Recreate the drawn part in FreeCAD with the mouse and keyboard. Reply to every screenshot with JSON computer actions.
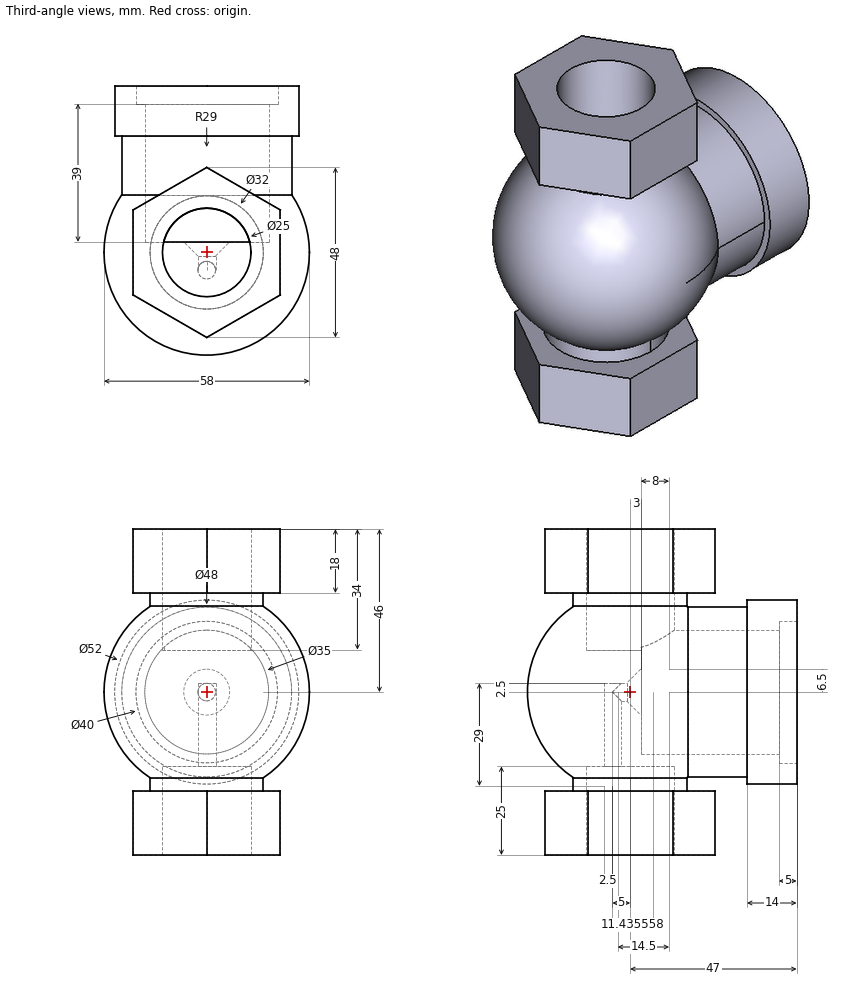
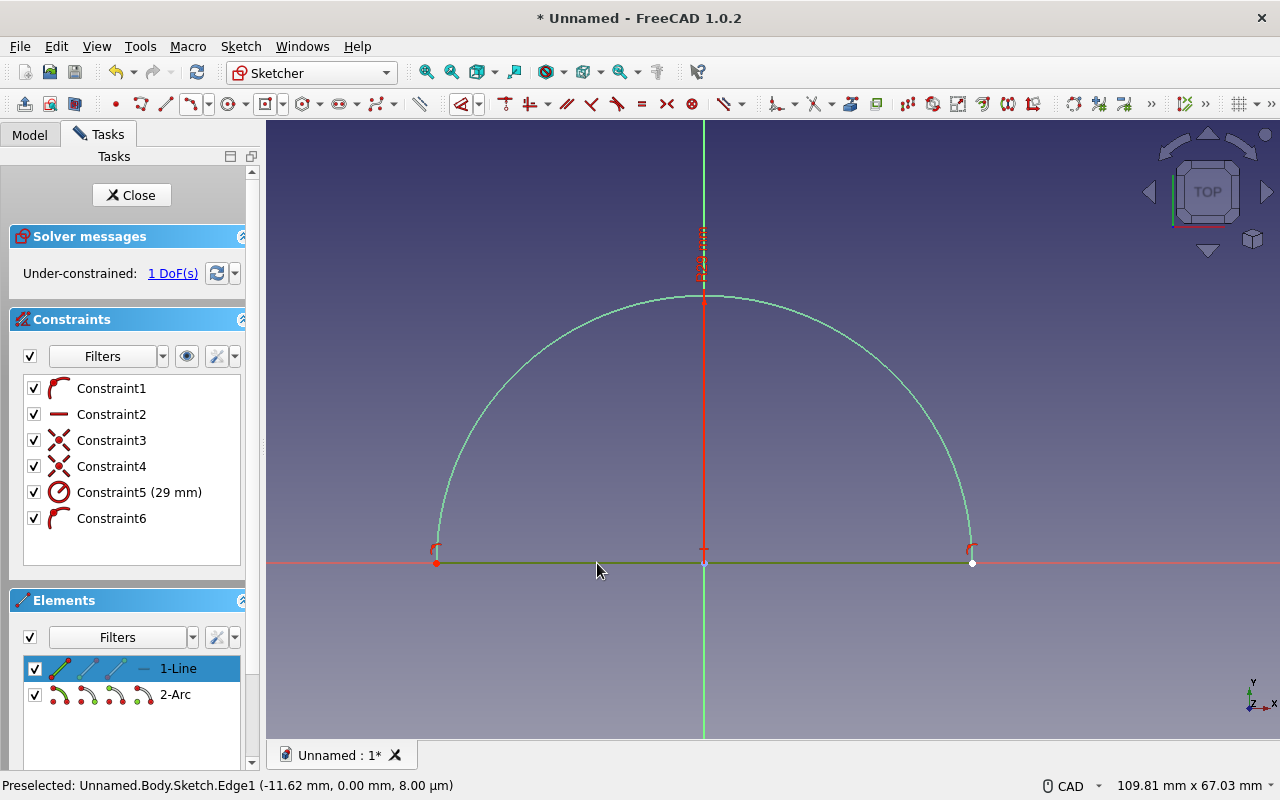
{"action": "key", "text": "l"}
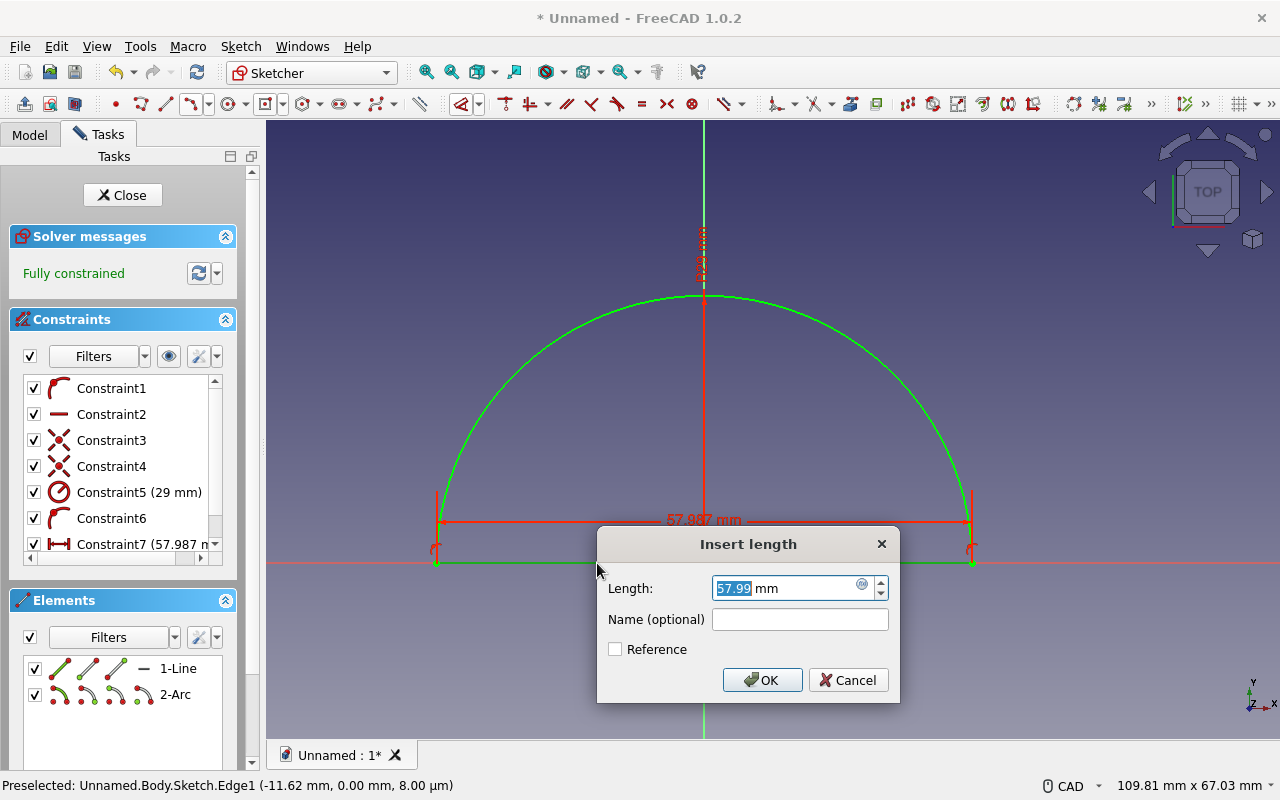
{"action": "type", "text": "58"}
{"action": "key", "text": "Return"}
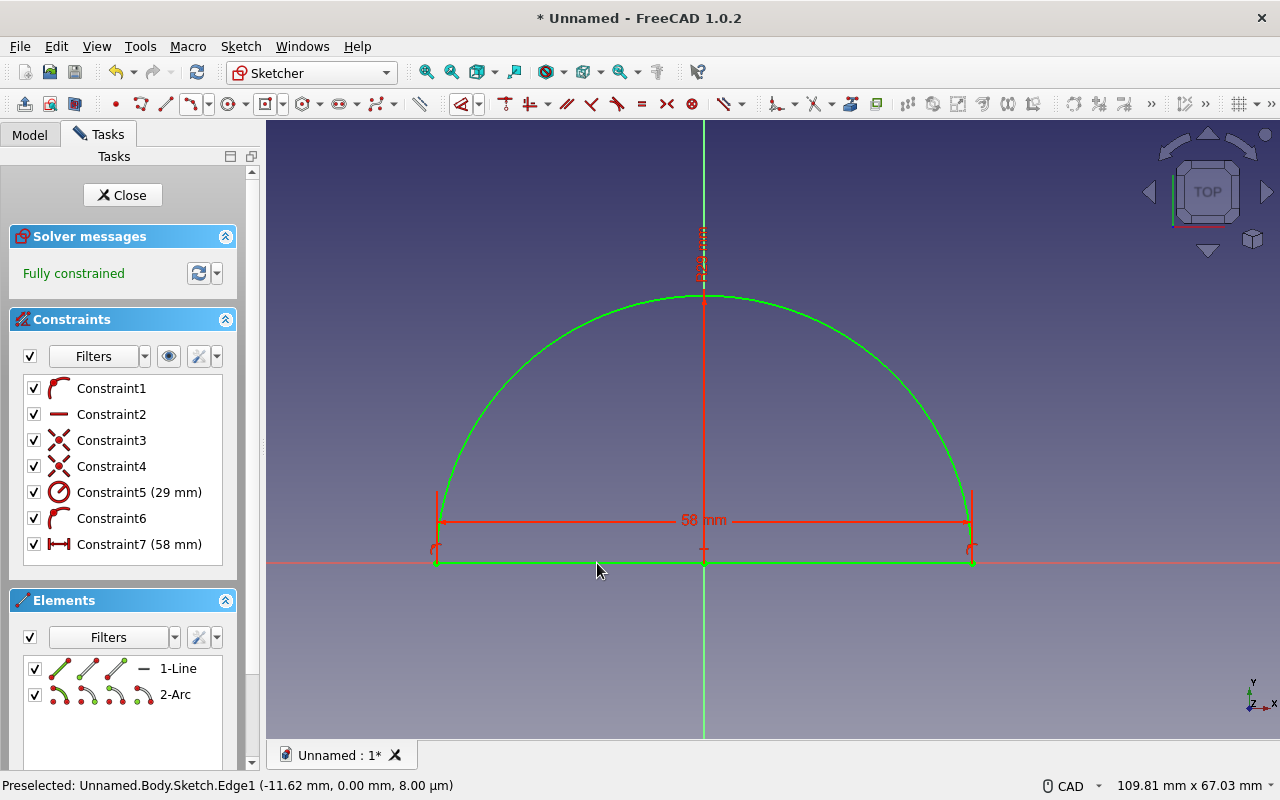
{"action": "left_click", "coordinate": [123, 195]}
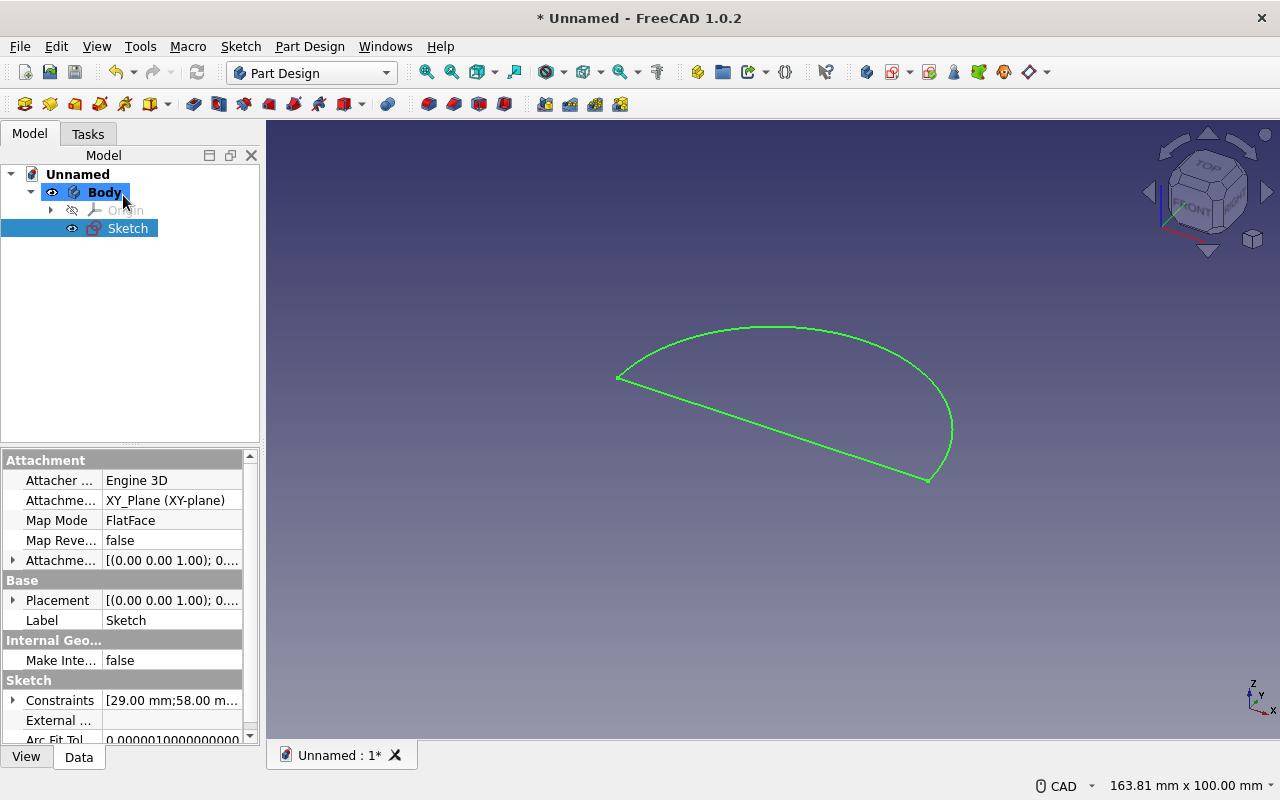
{"action": "left_click", "coordinate": [50, 104]}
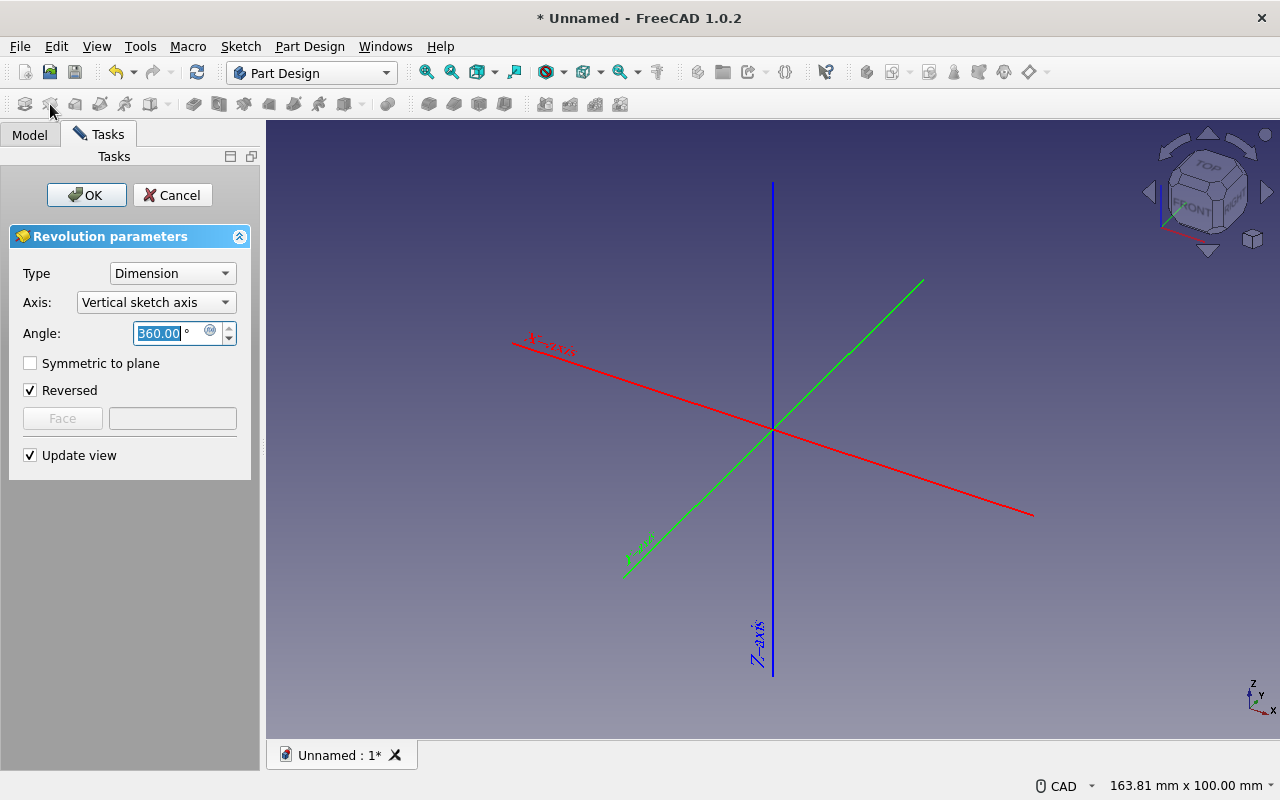
{"action": "left_click", "coordinate": [157, 302]}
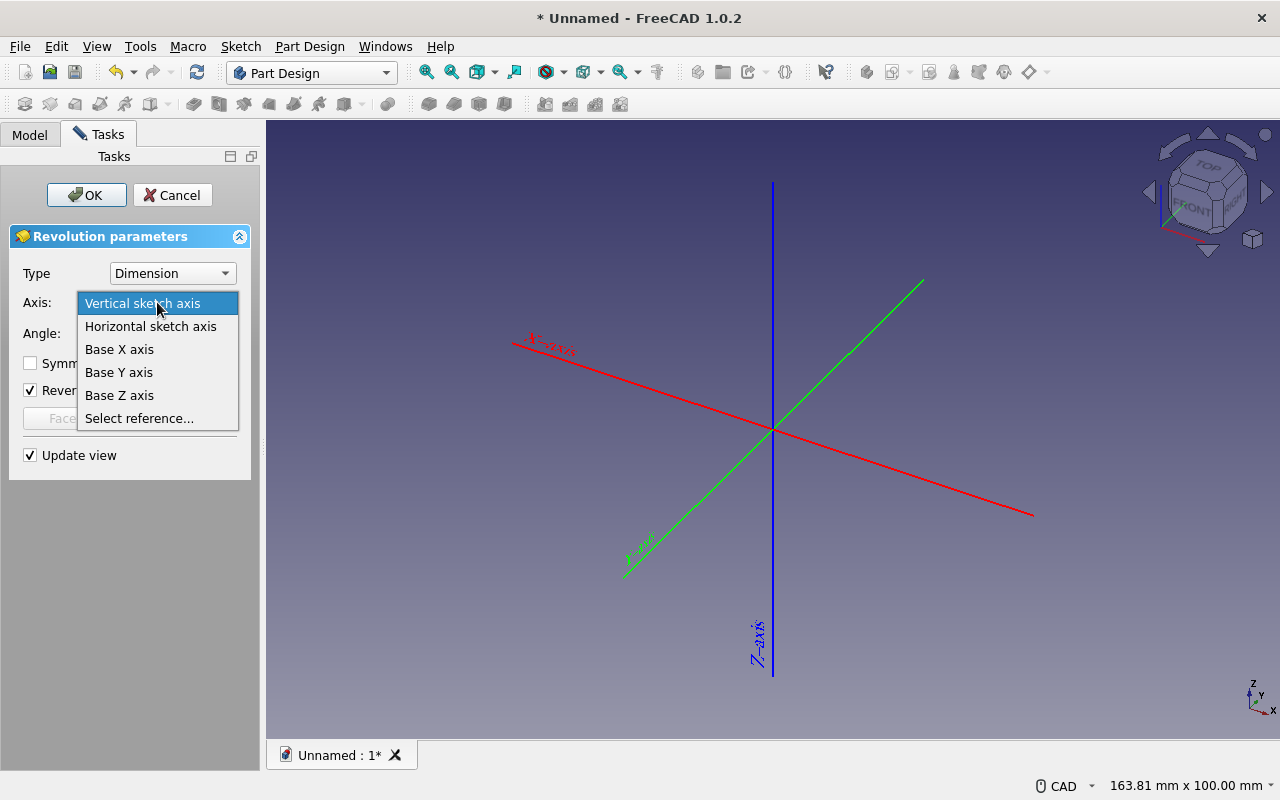
{"action": "left_click", "coordinate": [156, 326]}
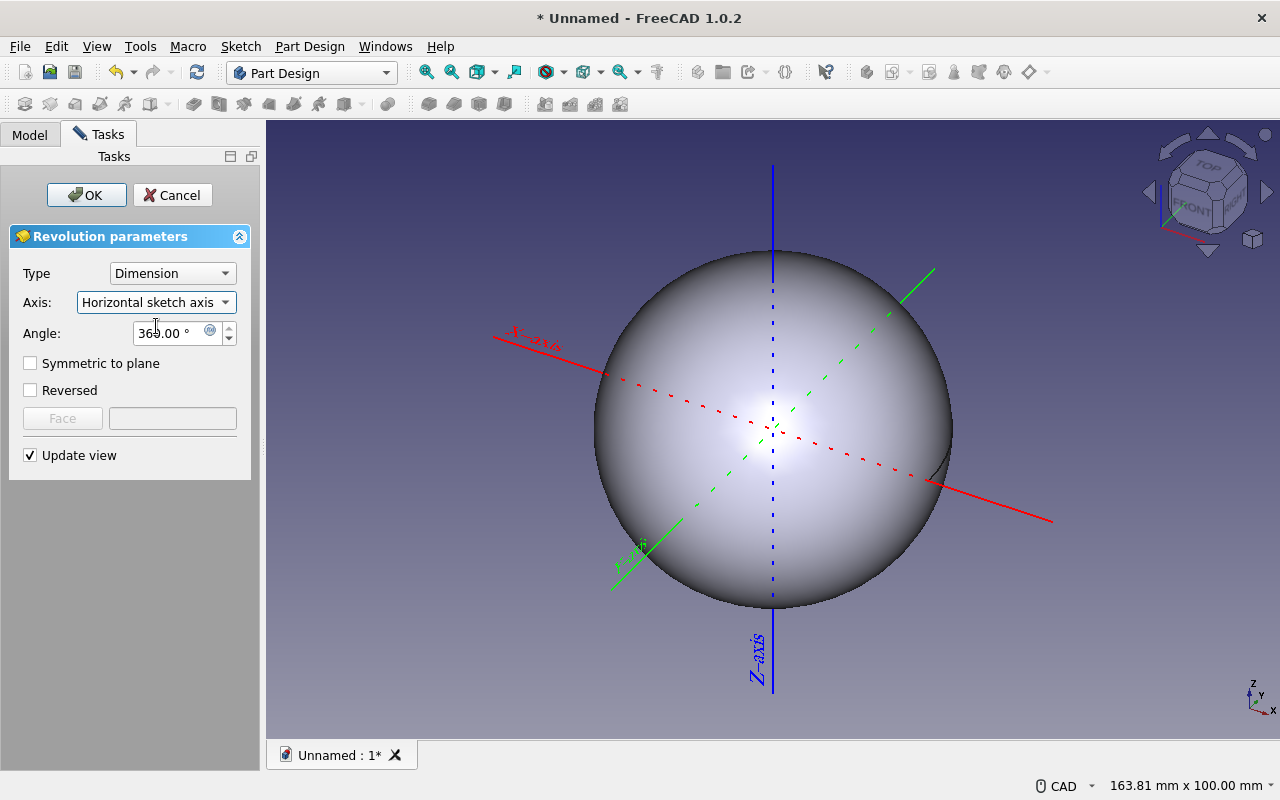
{"action": "left_click", "coordinate": [87, 195]}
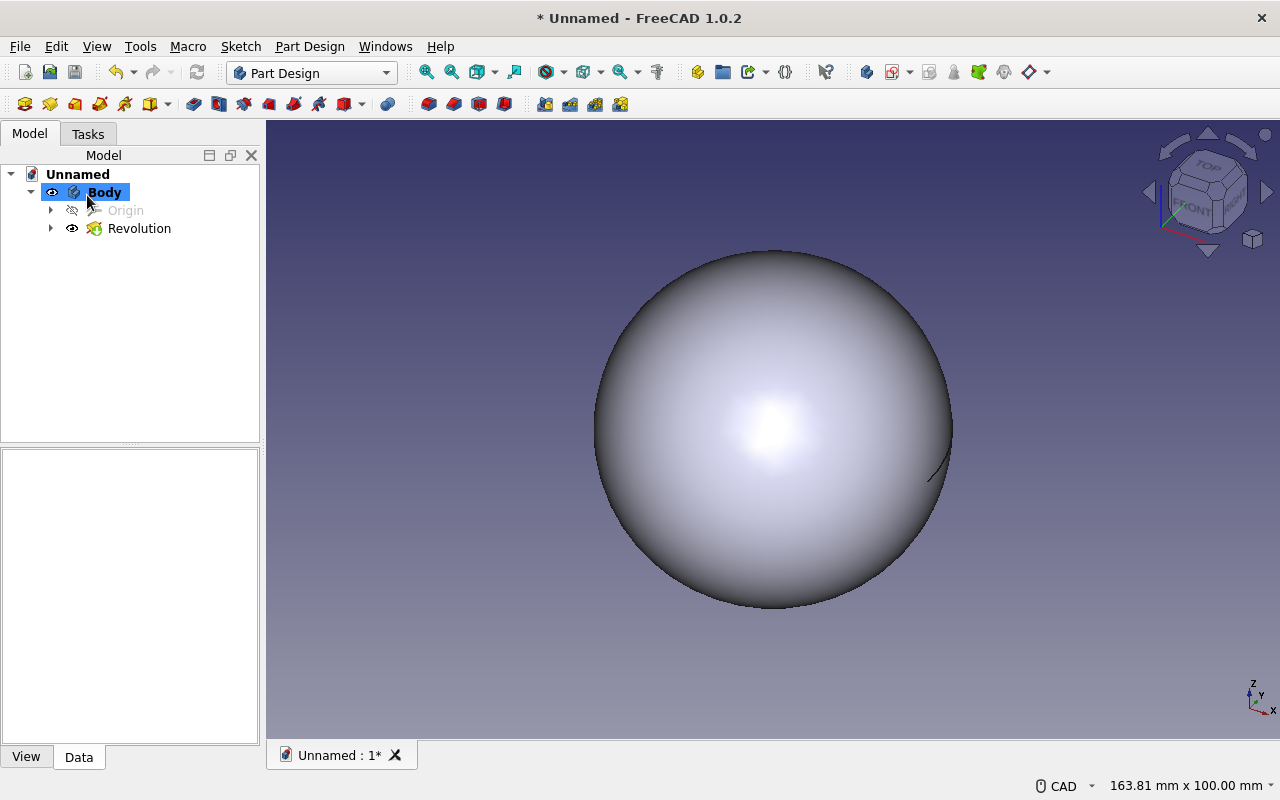
{"action": "left_click", "coordinate": [892, 72]}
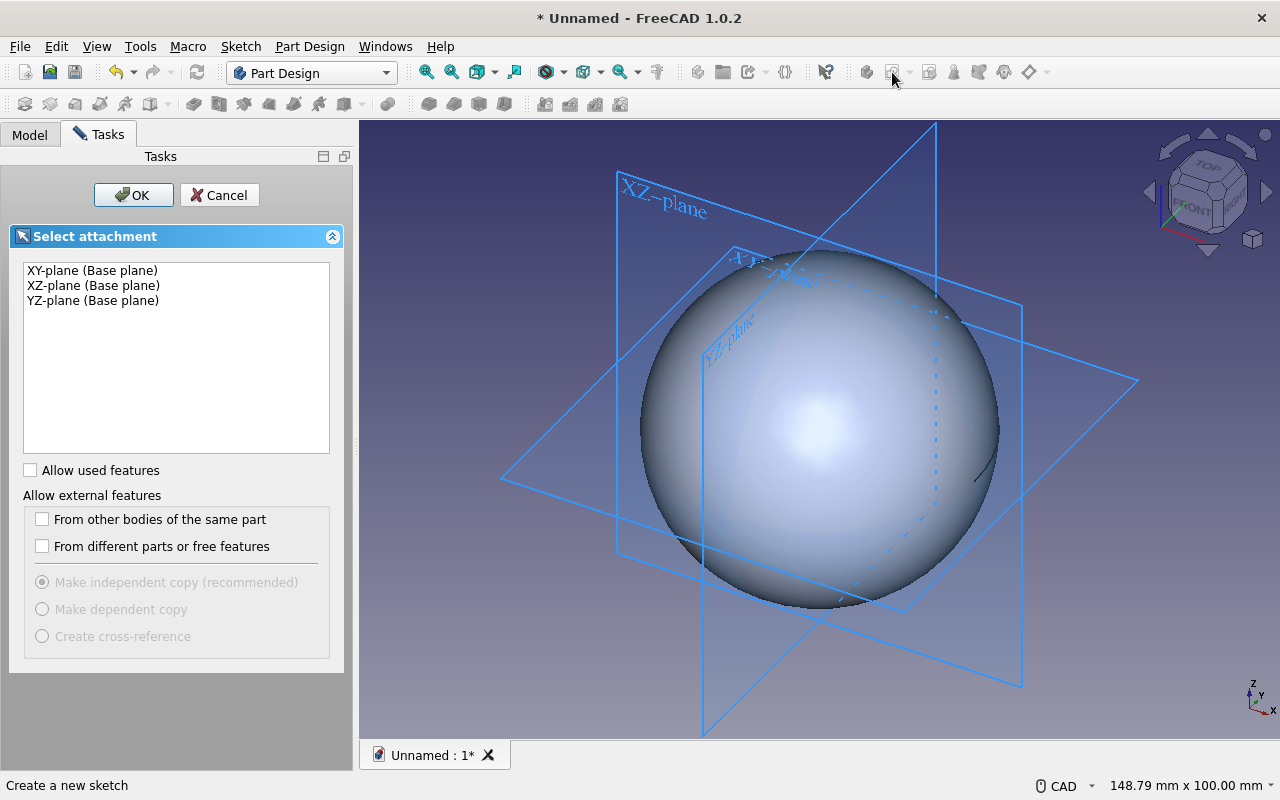
{"action": "left_click", "coordinate": [84, 286]}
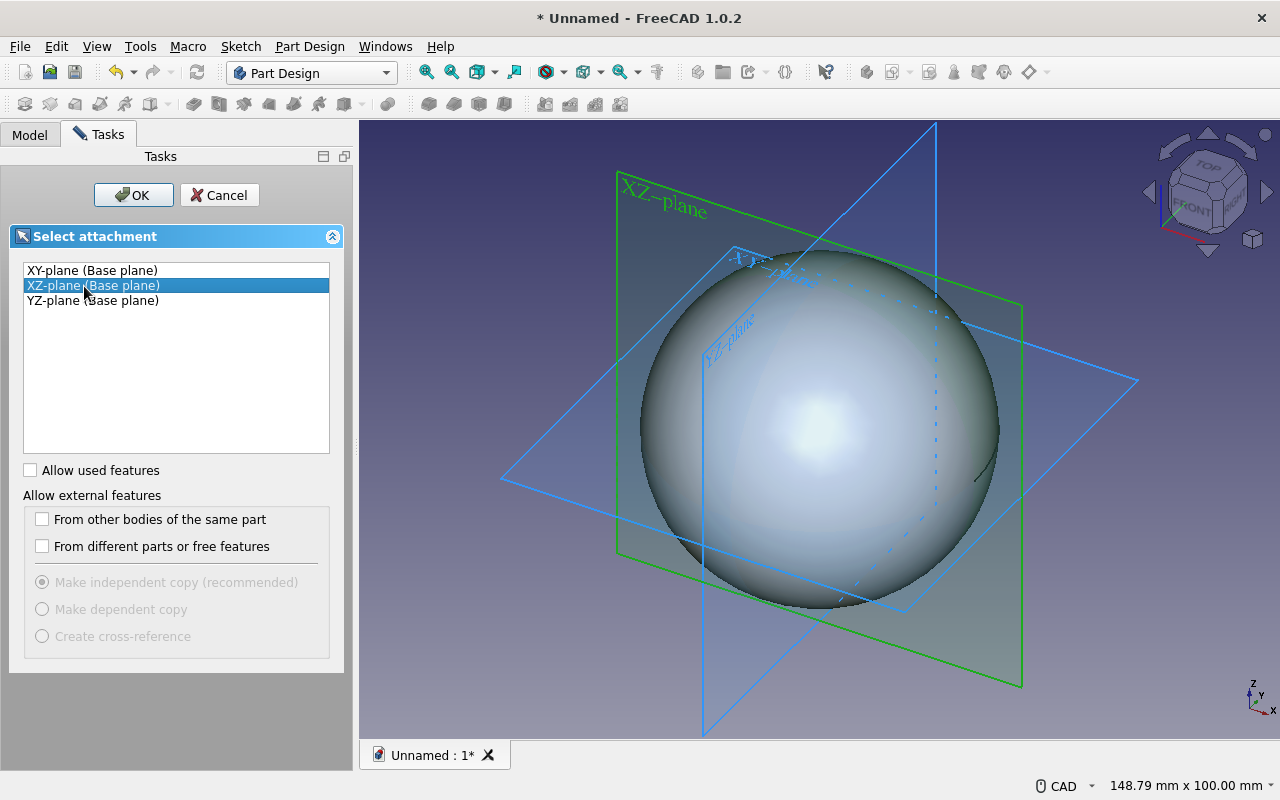
{"action": "left_click", "coordinate": [134, 195]}